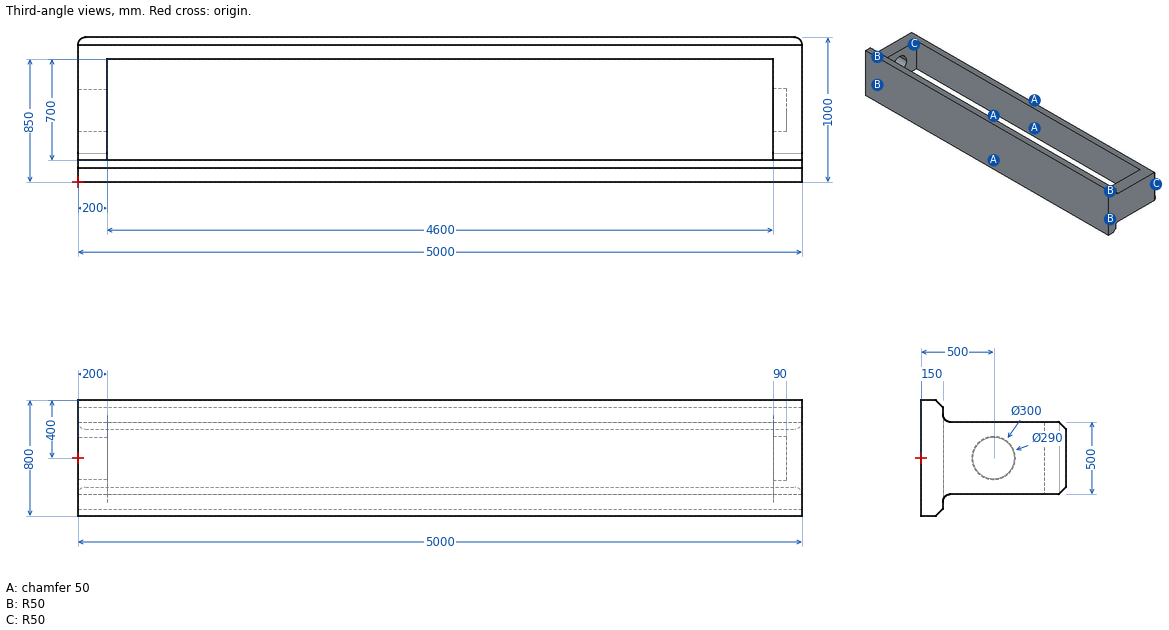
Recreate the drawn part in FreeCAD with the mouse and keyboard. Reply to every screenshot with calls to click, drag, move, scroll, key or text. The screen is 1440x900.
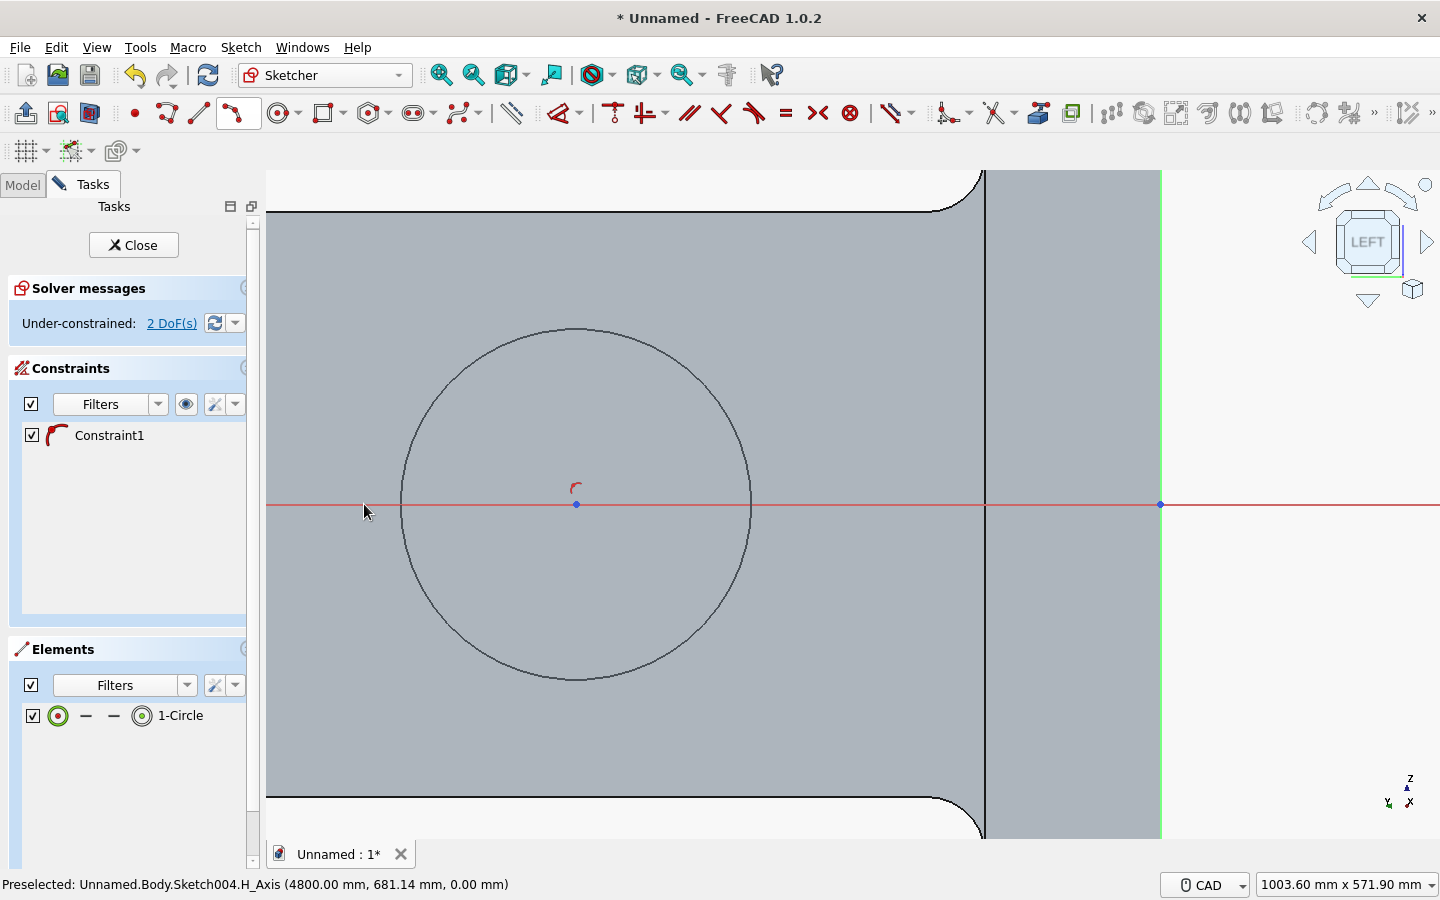
click(558, 114)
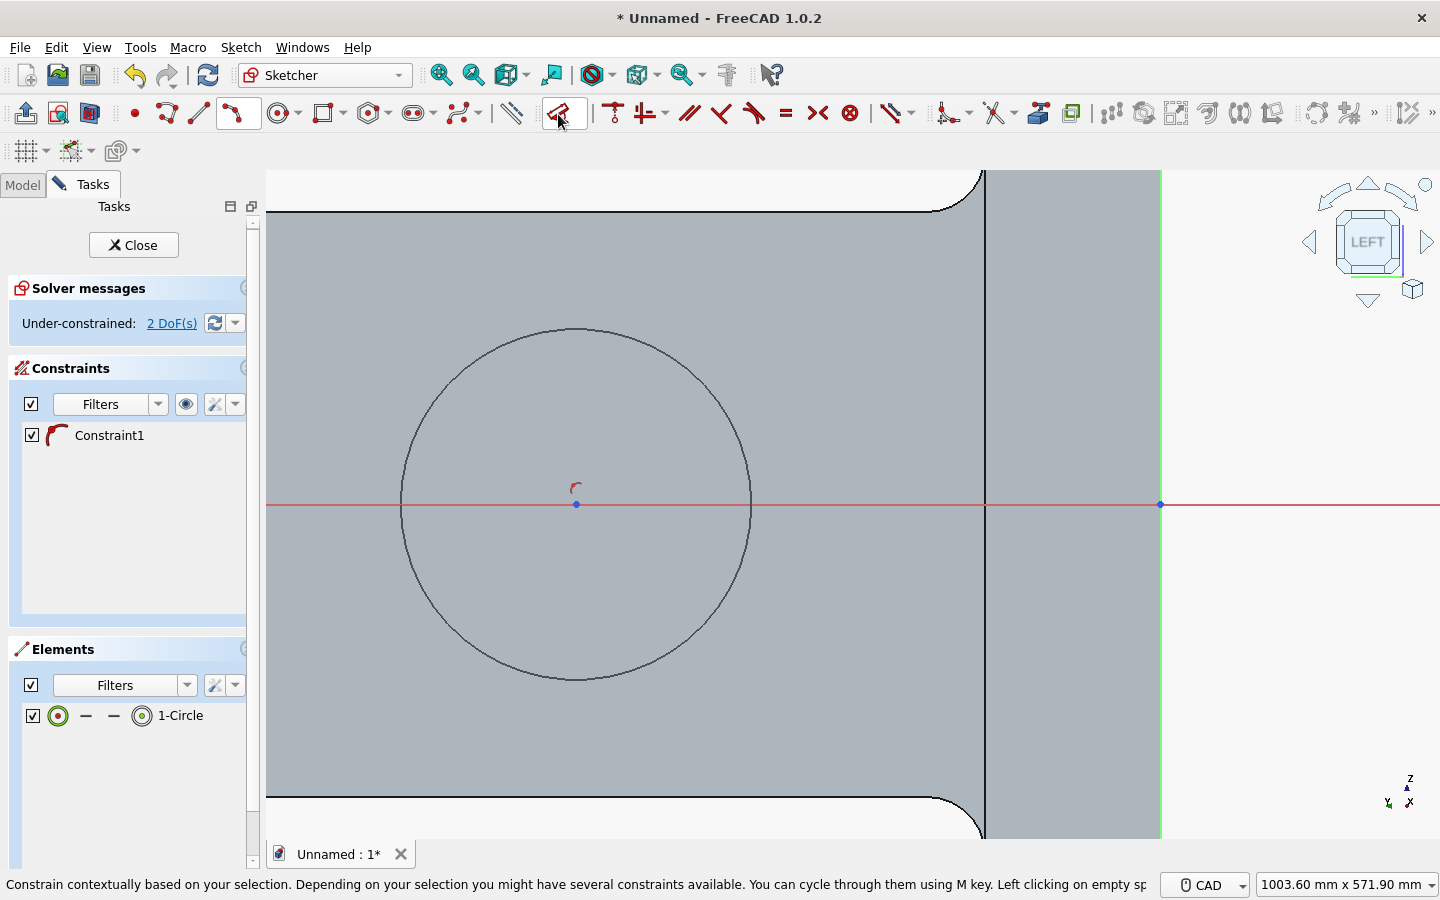
click(700, 380)
click(723, 357)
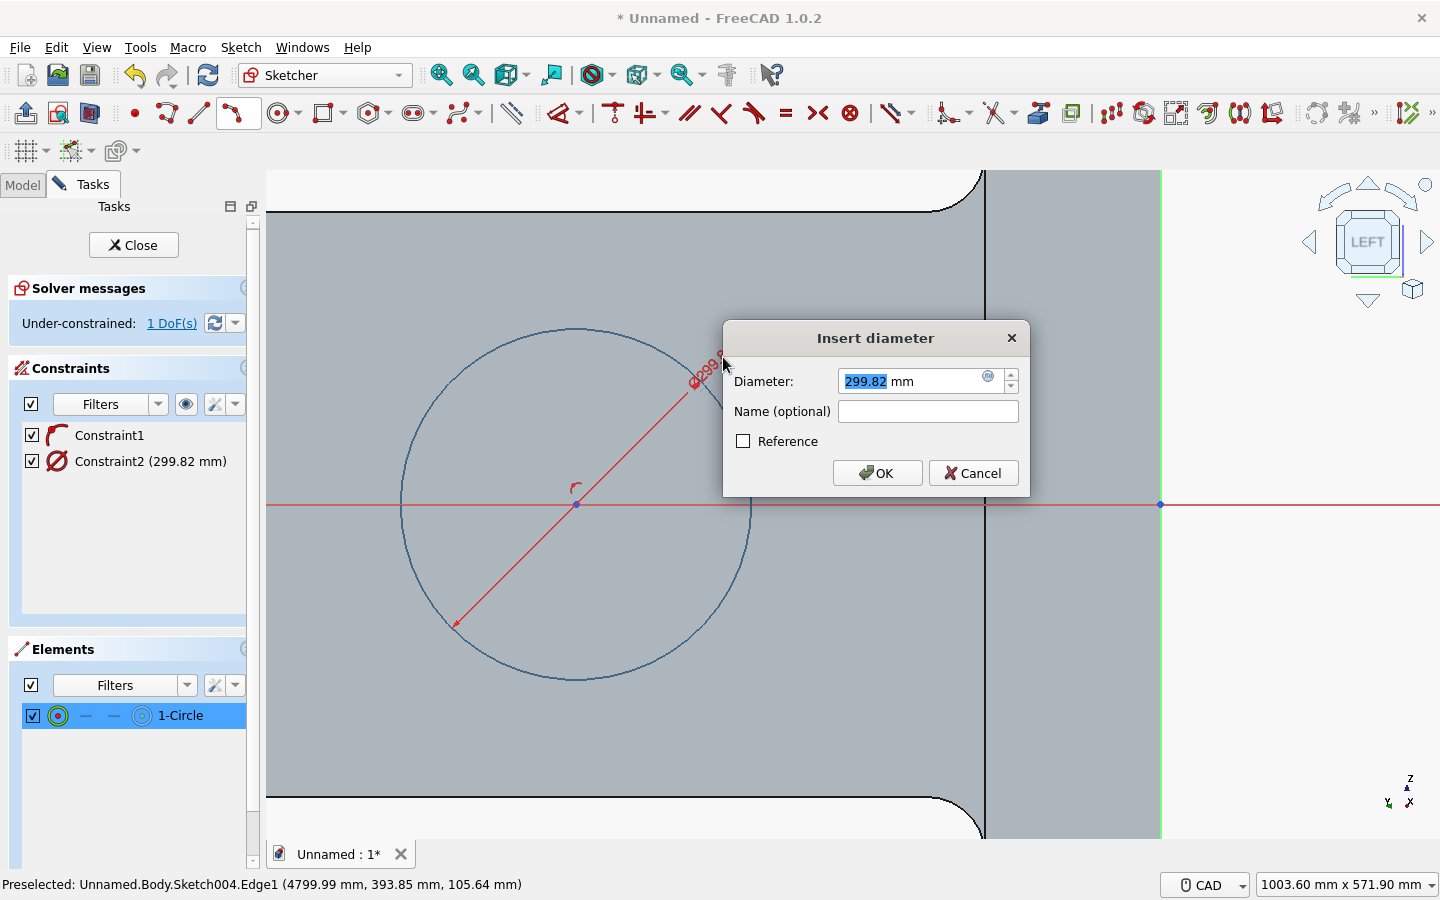
text(300)
key(Return)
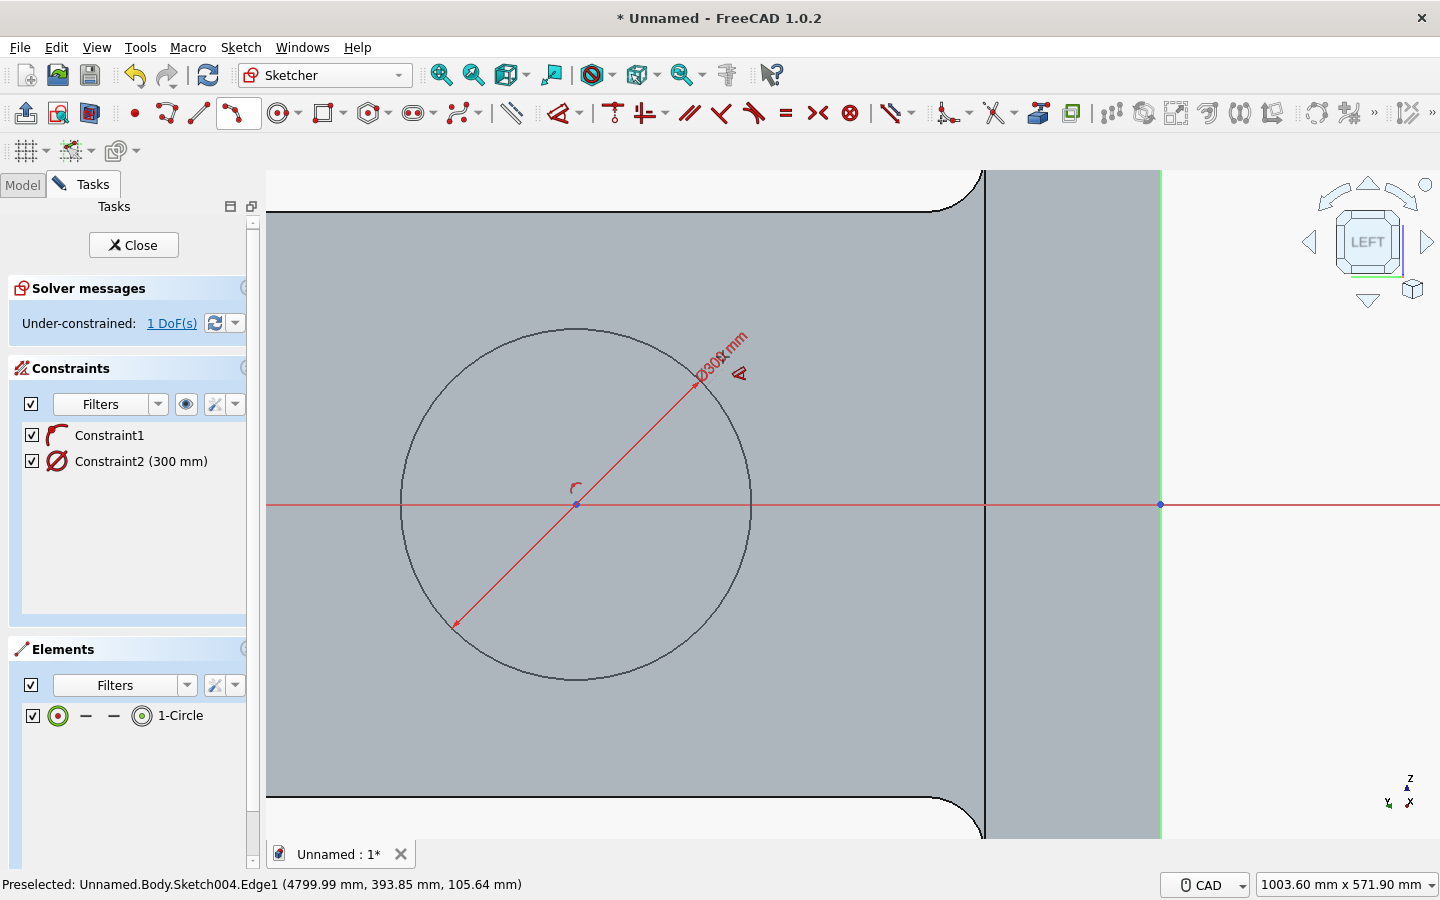
click(576, 504)
click(868, 538)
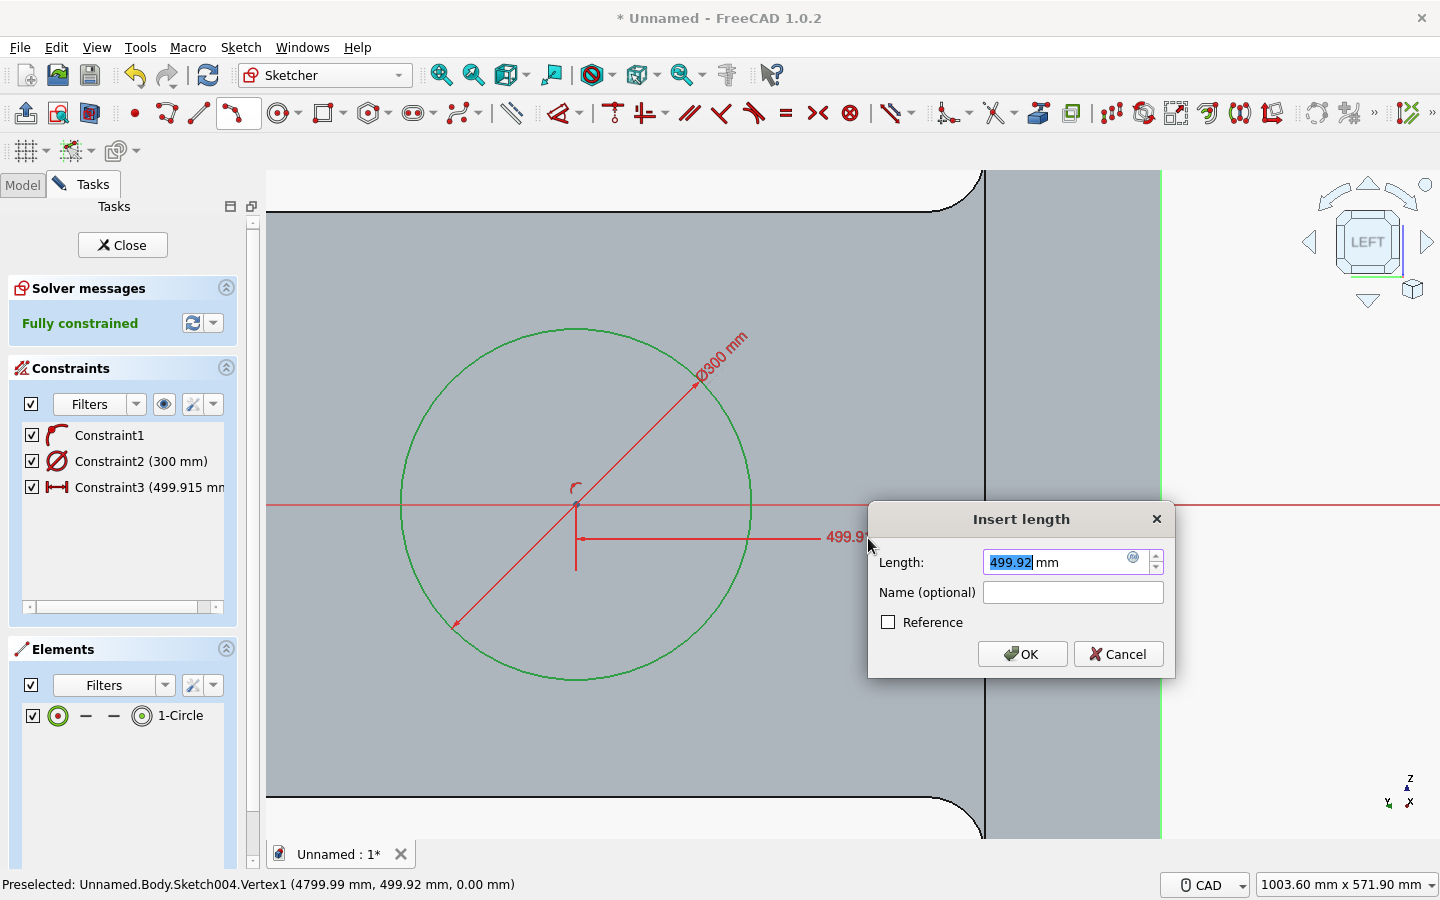
text(500)
key(Return)
key(Escape)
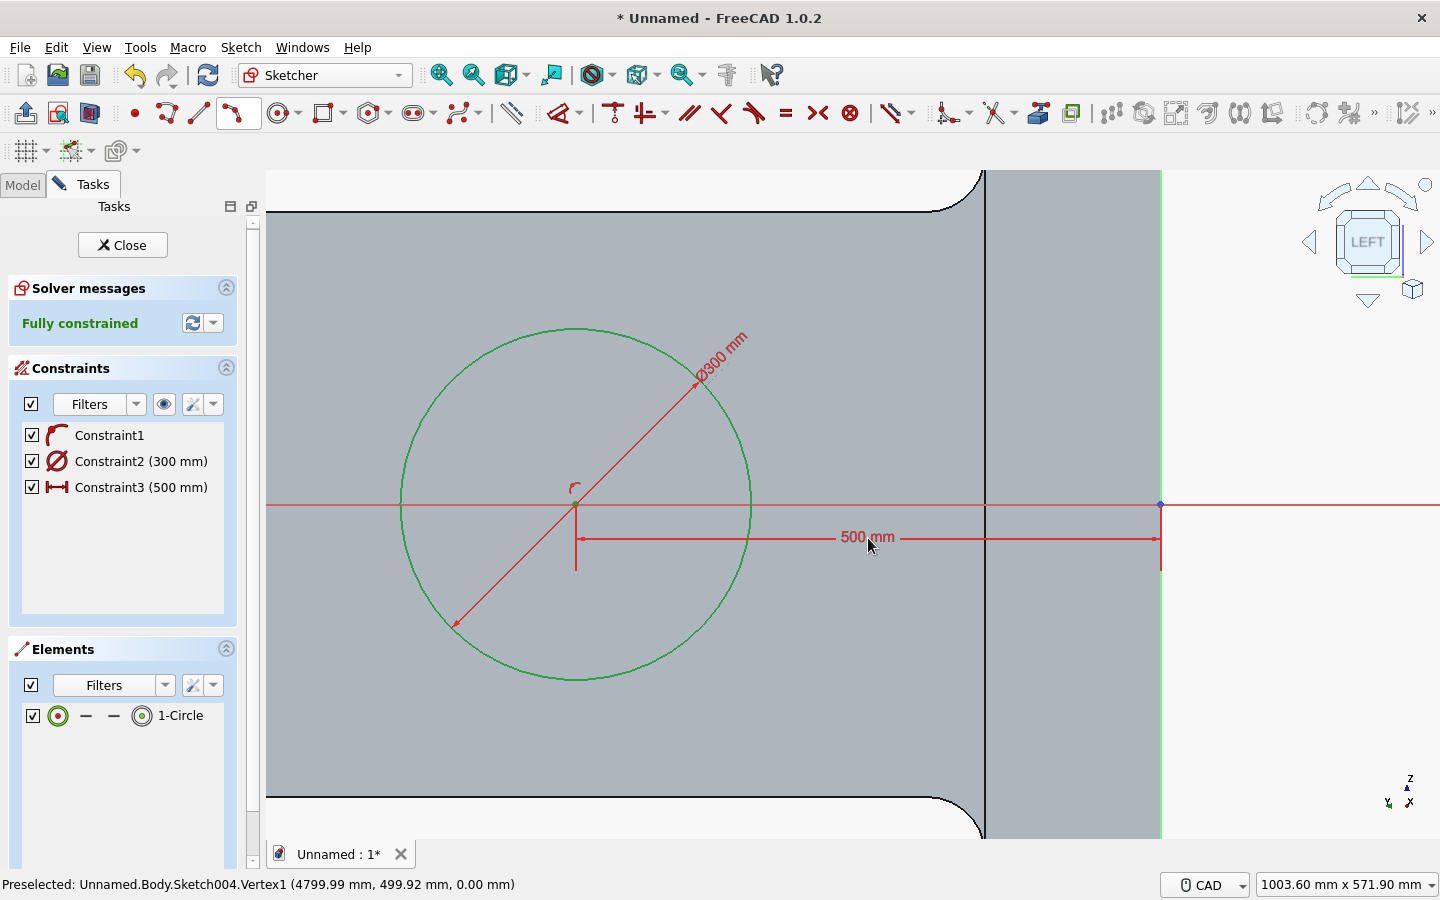
click(123, 245)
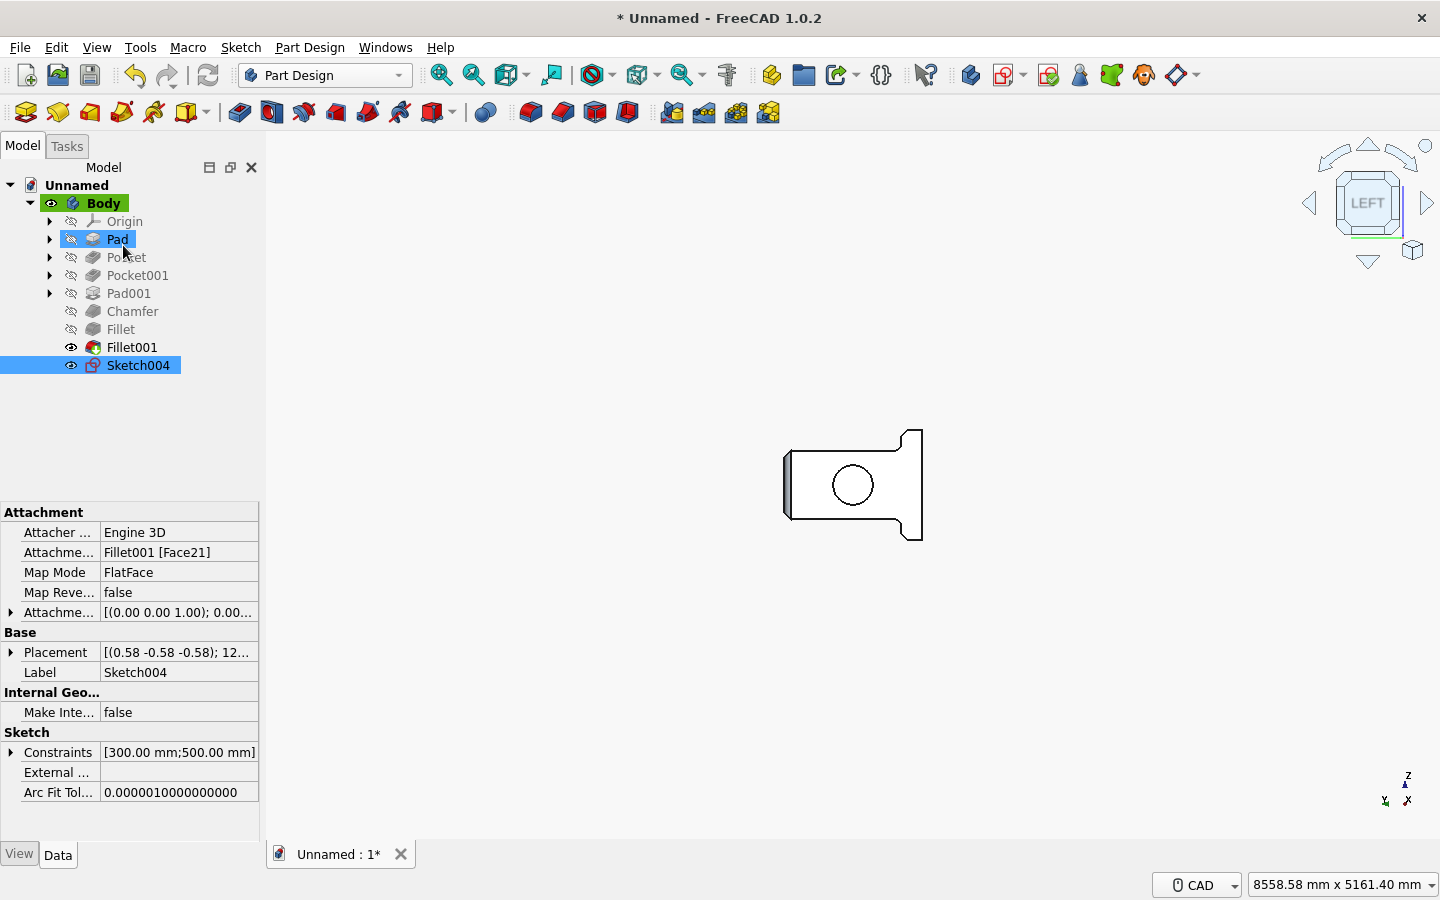
click(240, 112)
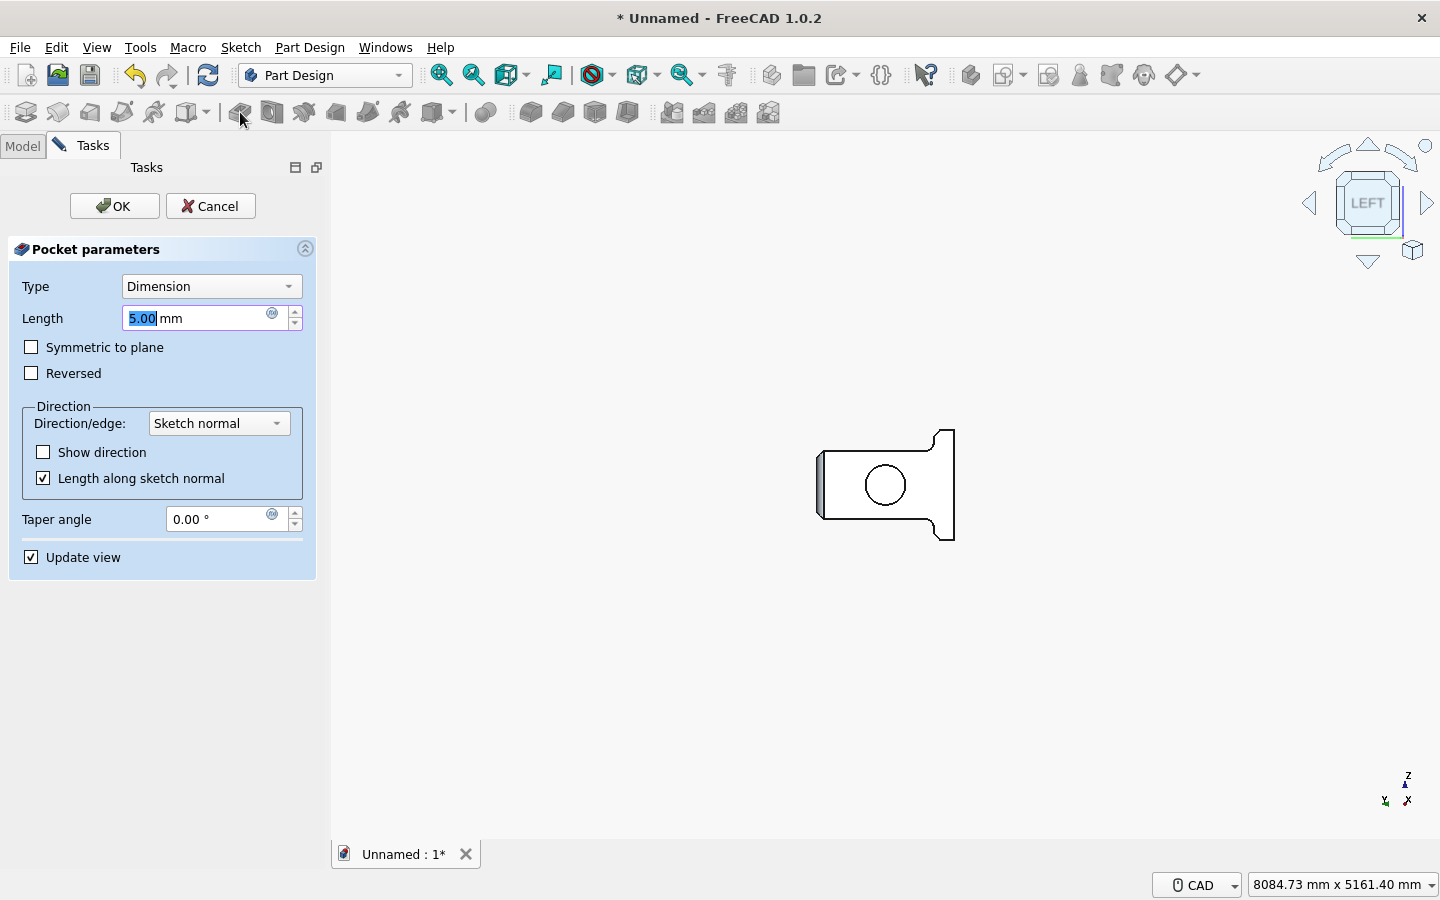
text(90)
key(Tab)